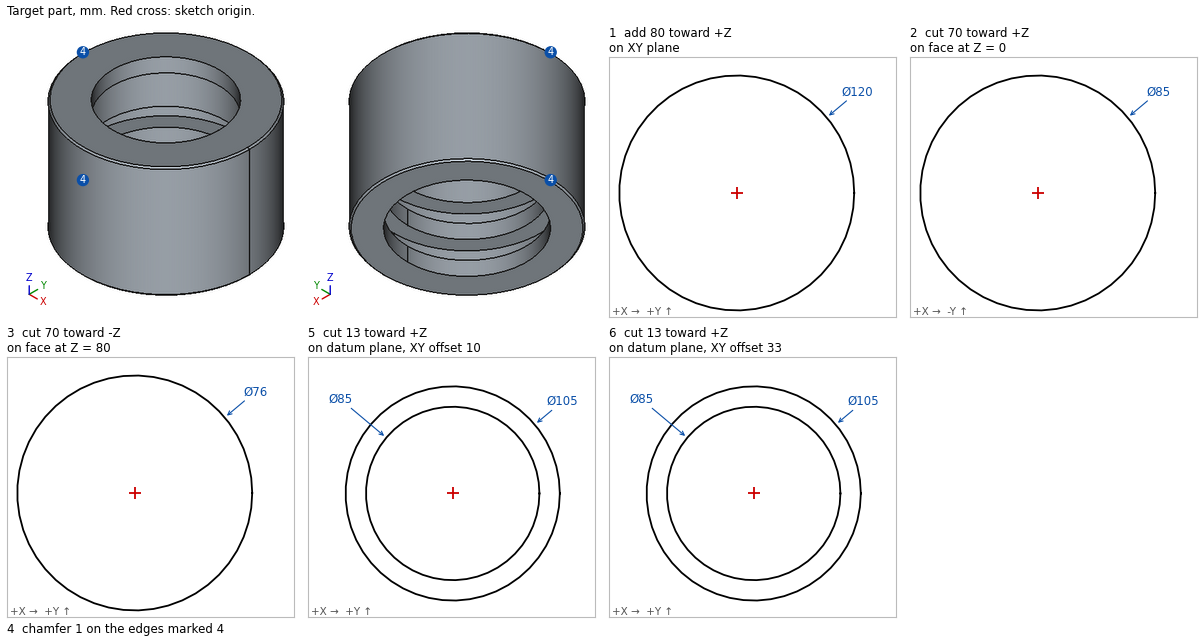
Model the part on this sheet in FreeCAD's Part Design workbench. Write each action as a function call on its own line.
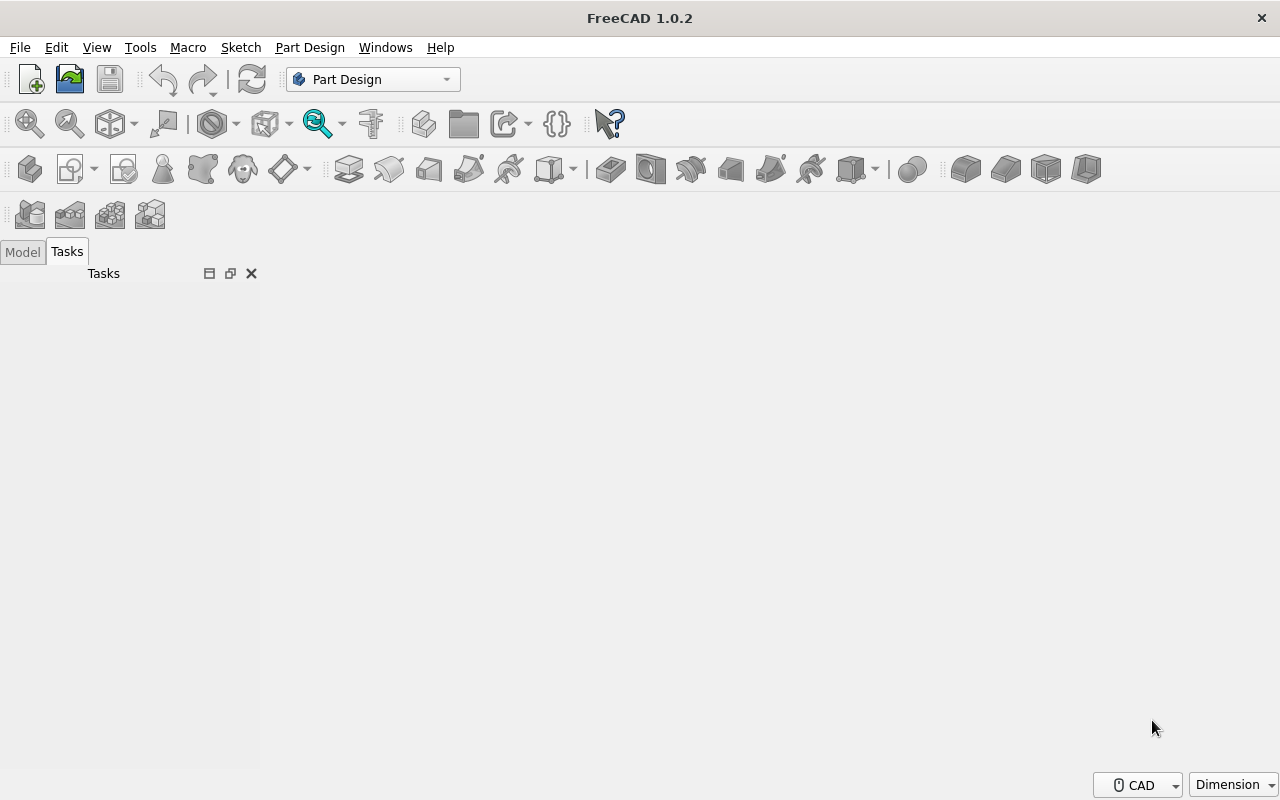
click(30, 80)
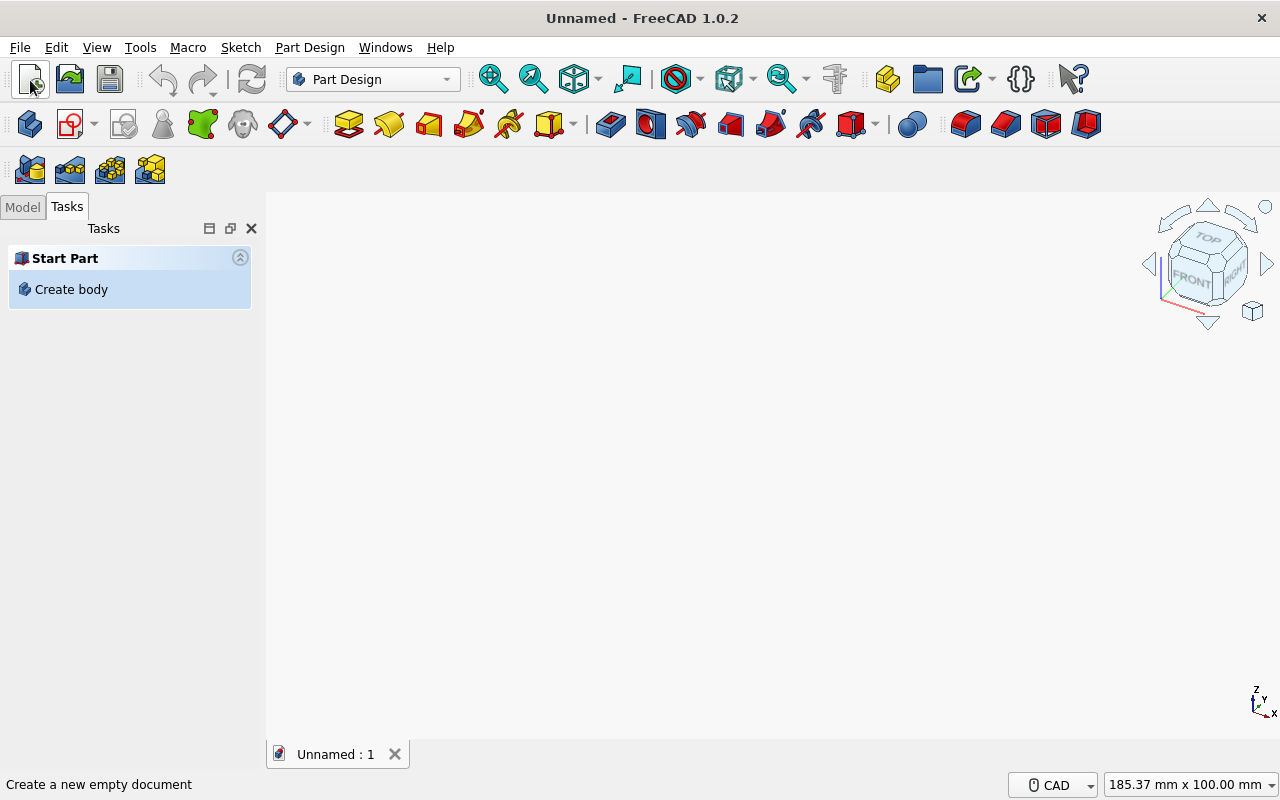
click(70, 124)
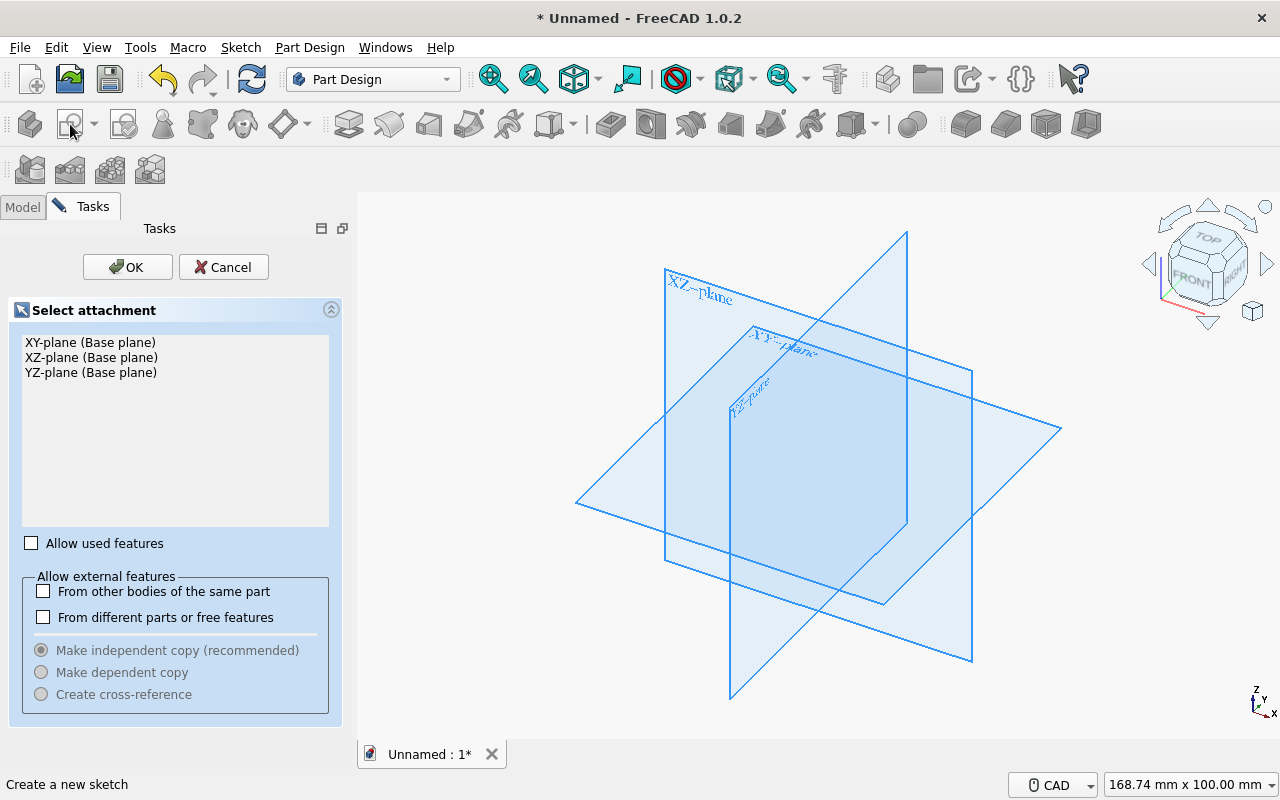
click(82, 342)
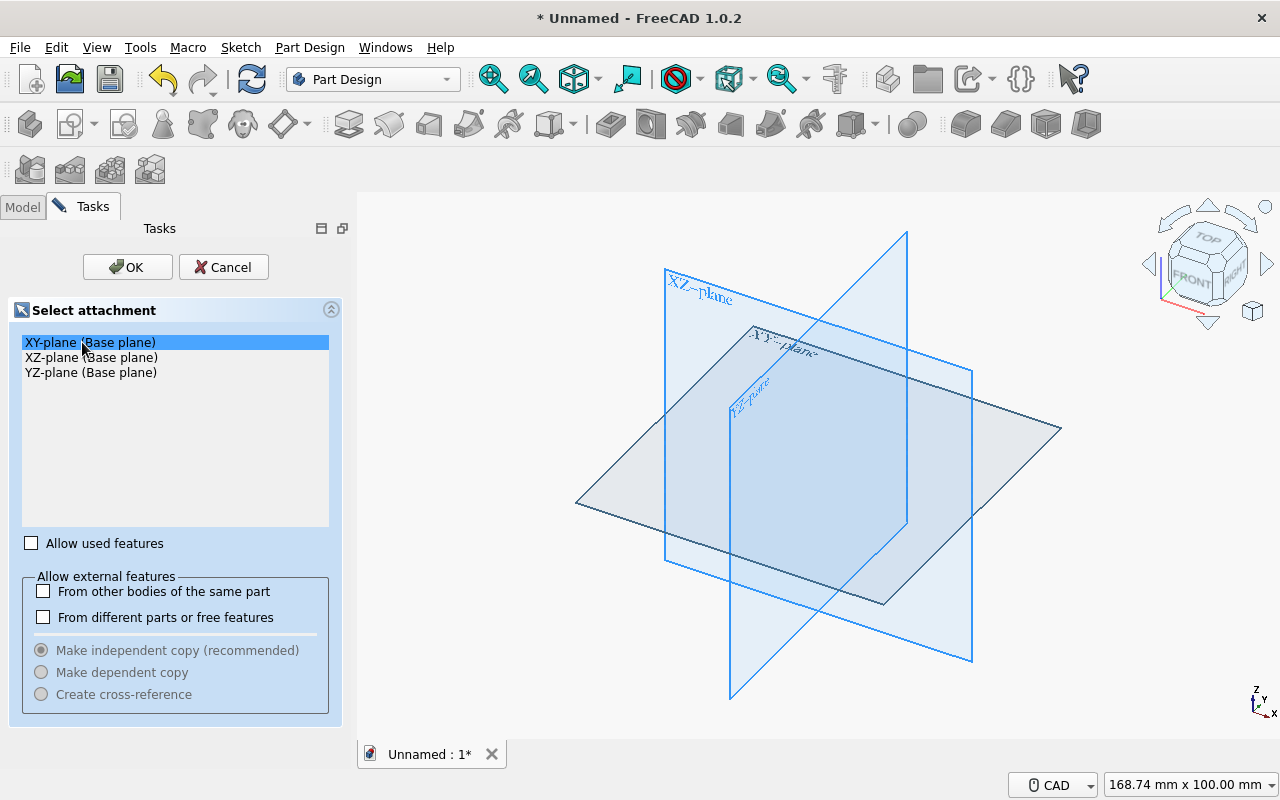
click(128, 267)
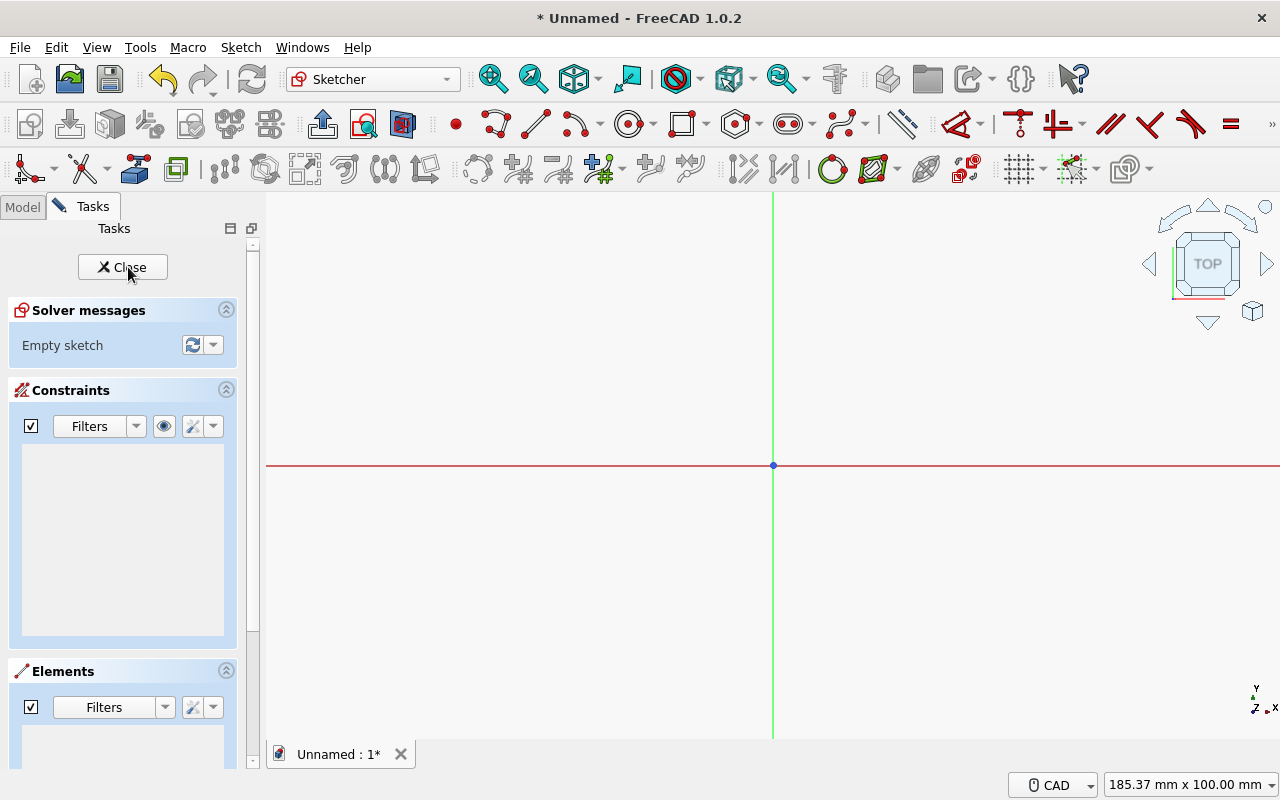
scroll(621, 466, down, 3)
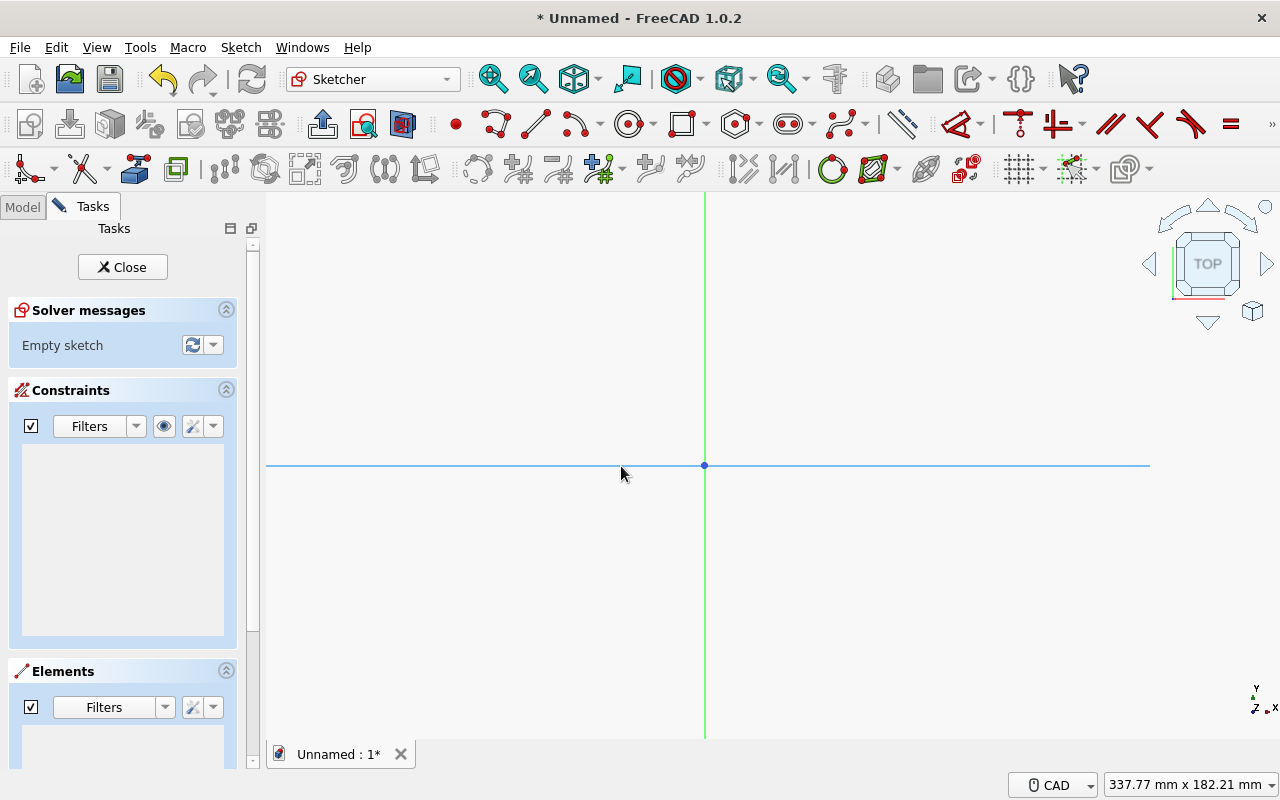
click(630, 124)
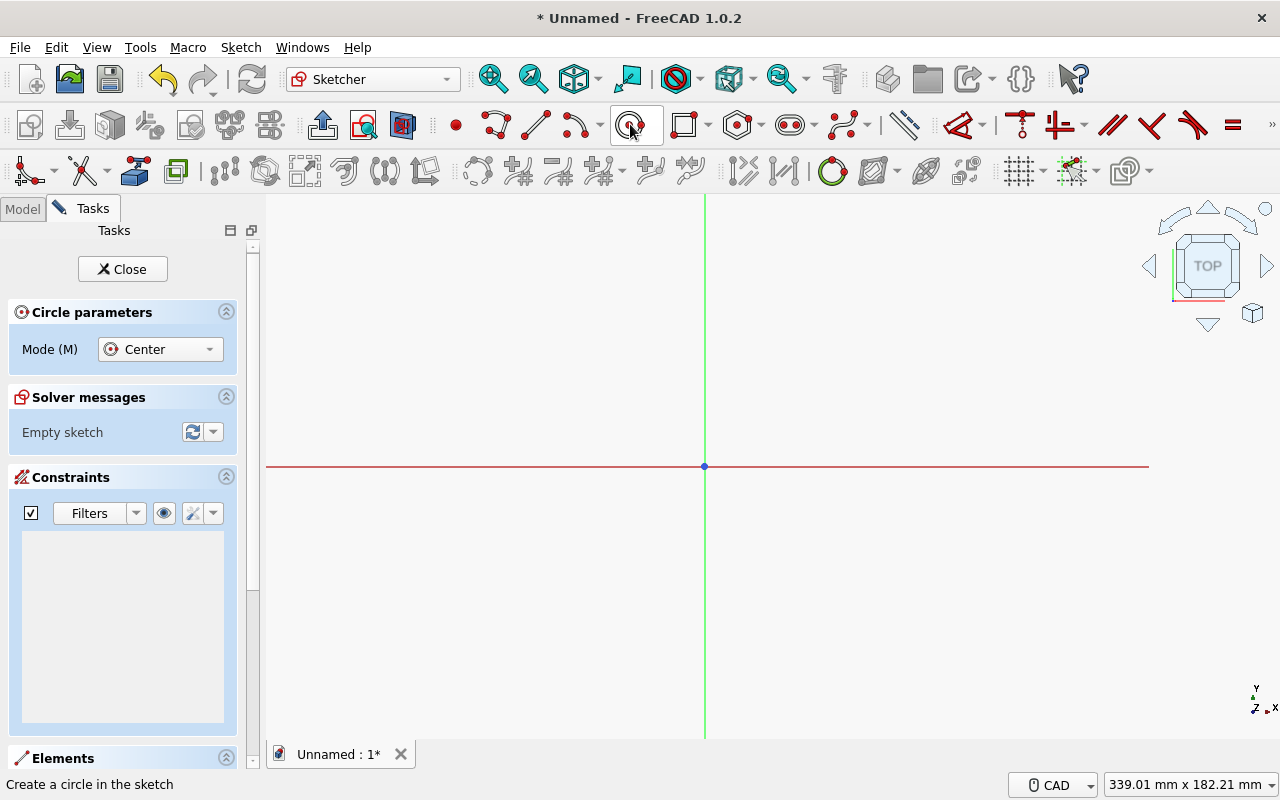
click(705, 467)
click(832, 340)
key(Escape)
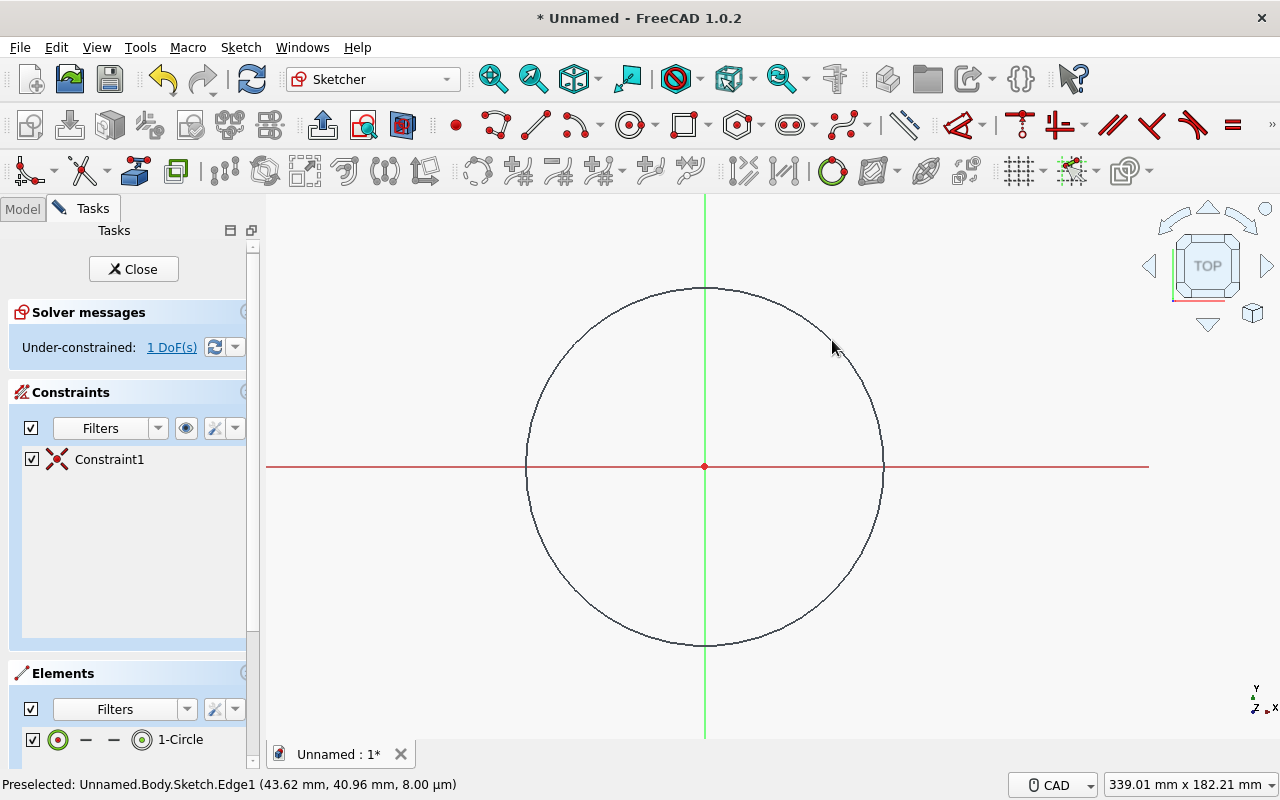
click(831, 340)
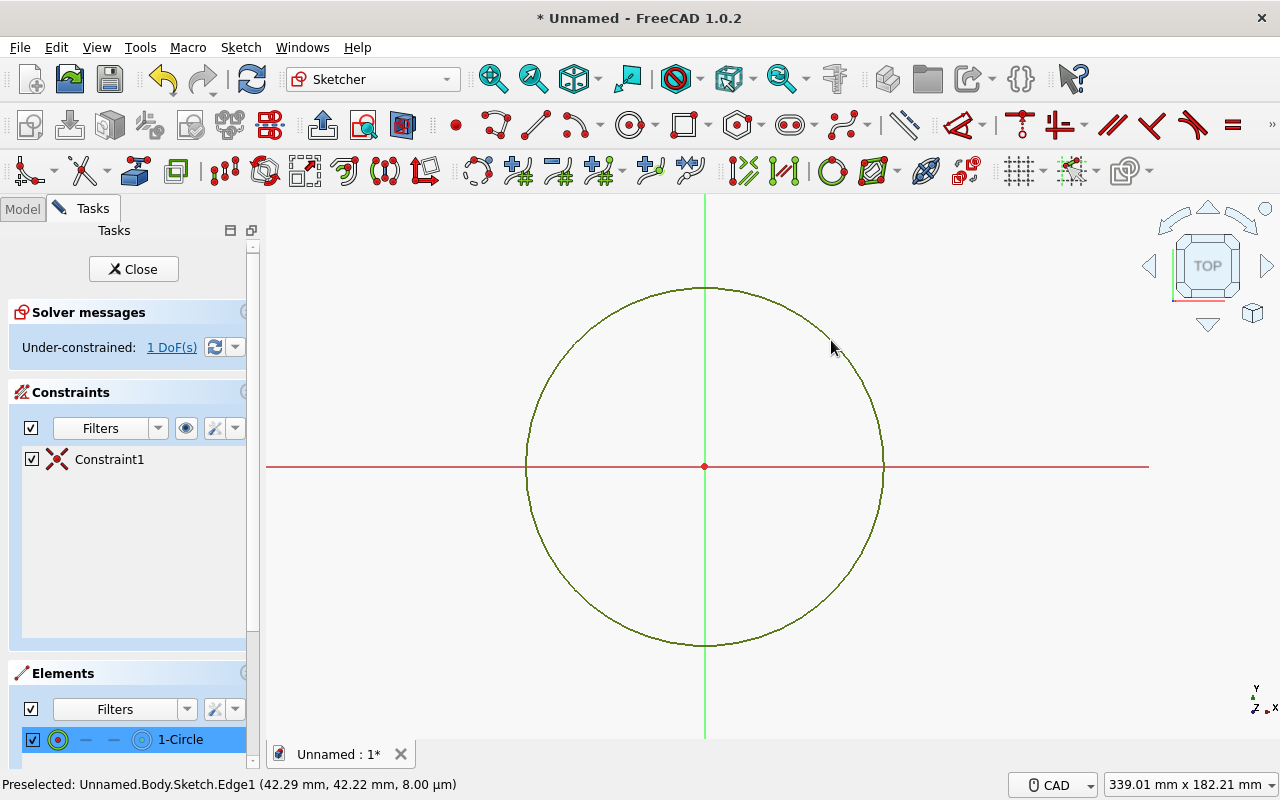
key(k)
key(o)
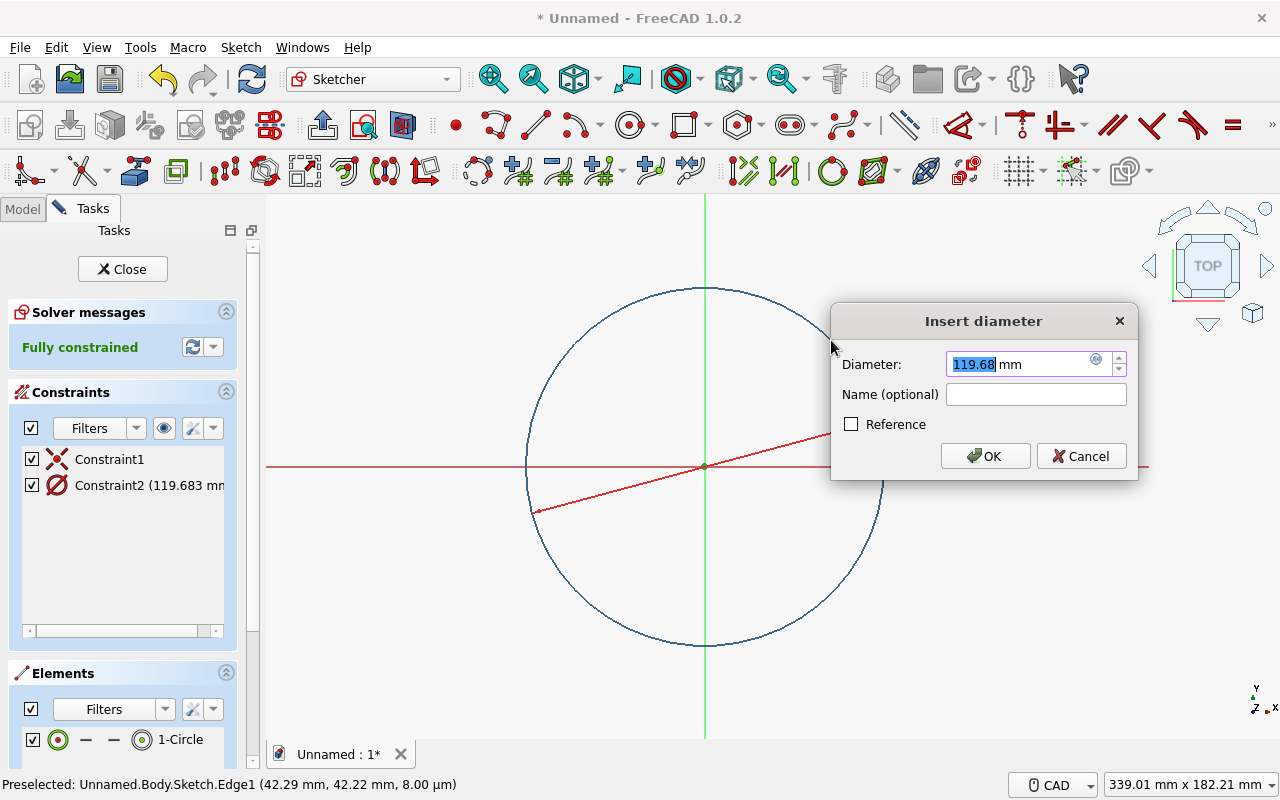
text(120)
key(Return)